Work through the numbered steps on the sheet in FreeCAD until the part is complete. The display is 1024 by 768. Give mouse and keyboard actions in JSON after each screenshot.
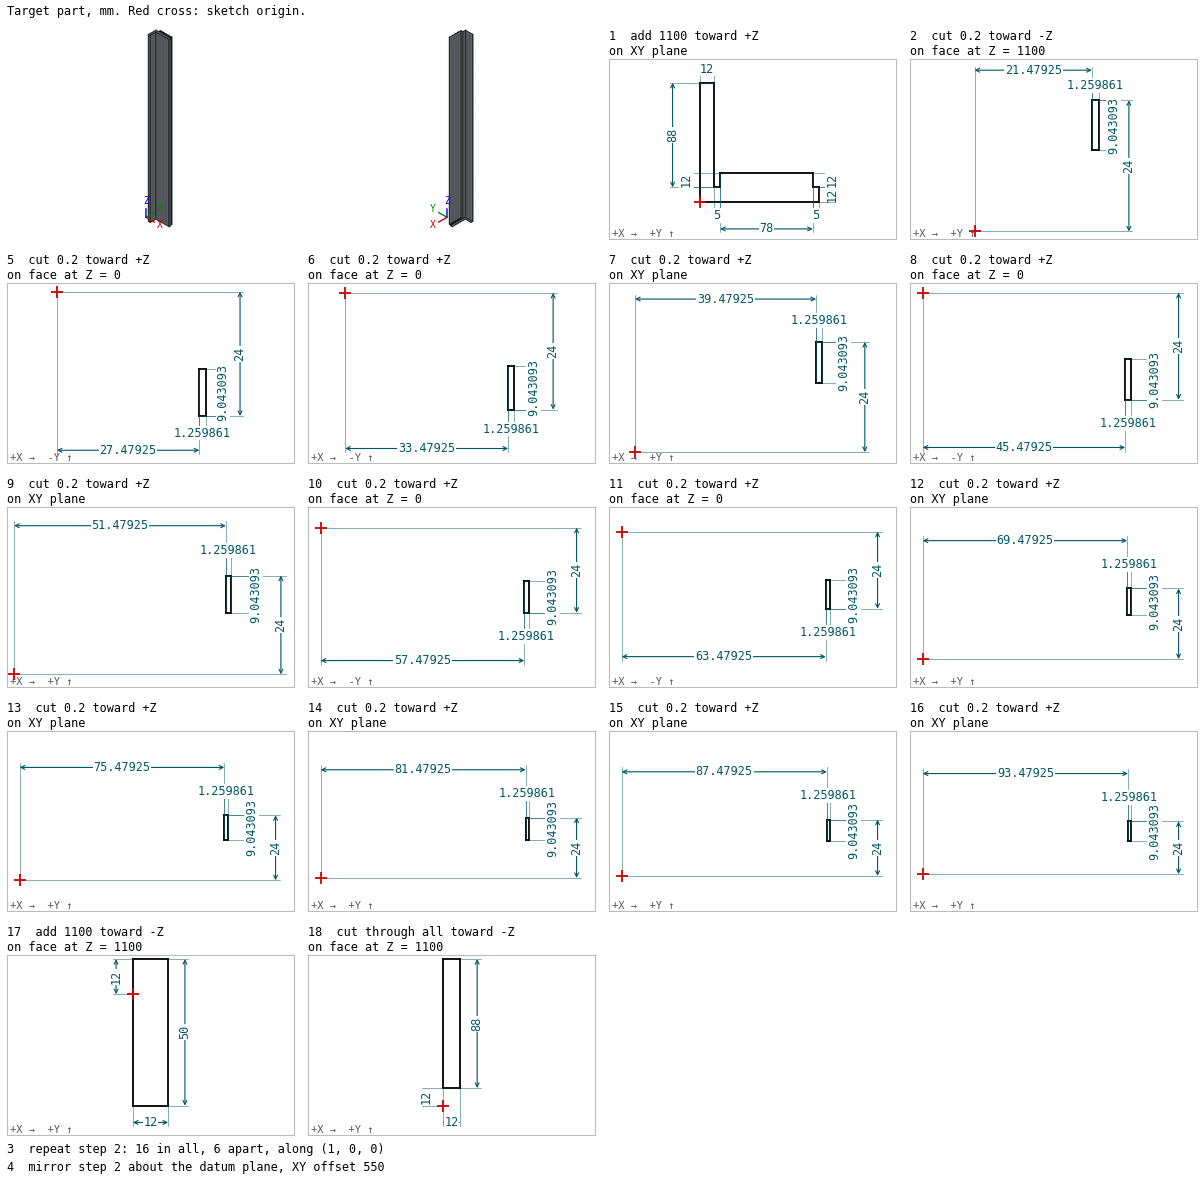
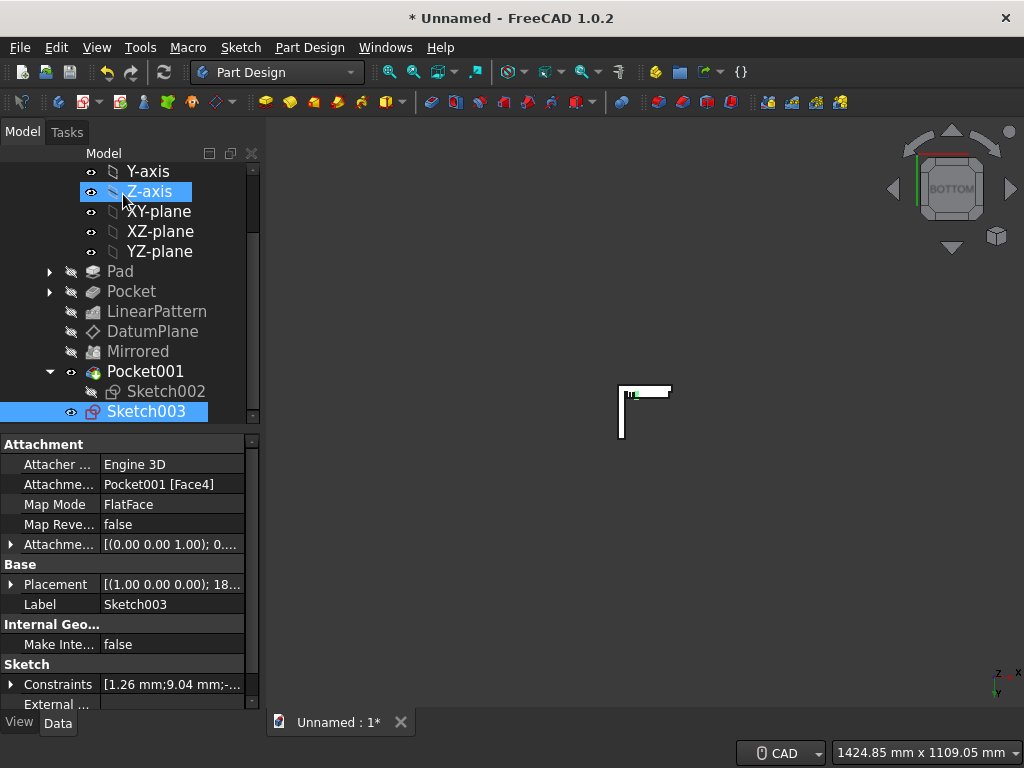
{"action": "left_click", "coordinate": [432, 102]}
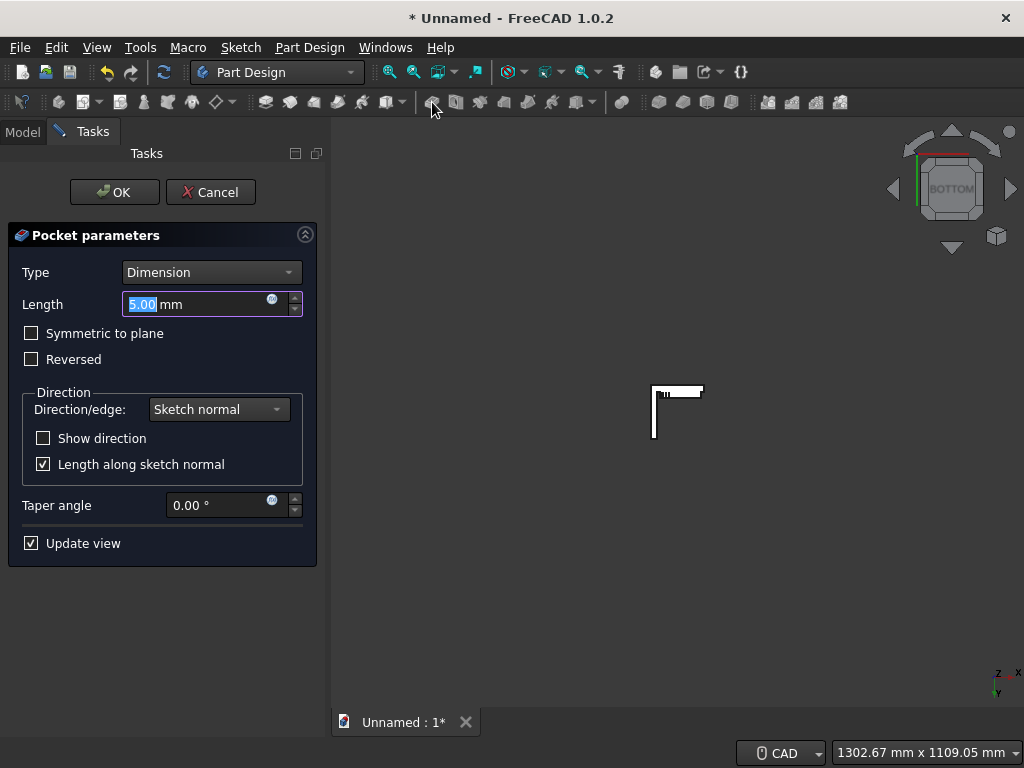
{"action": "type", "text": "0.2"}
{"action": "key", "text": "Tab"}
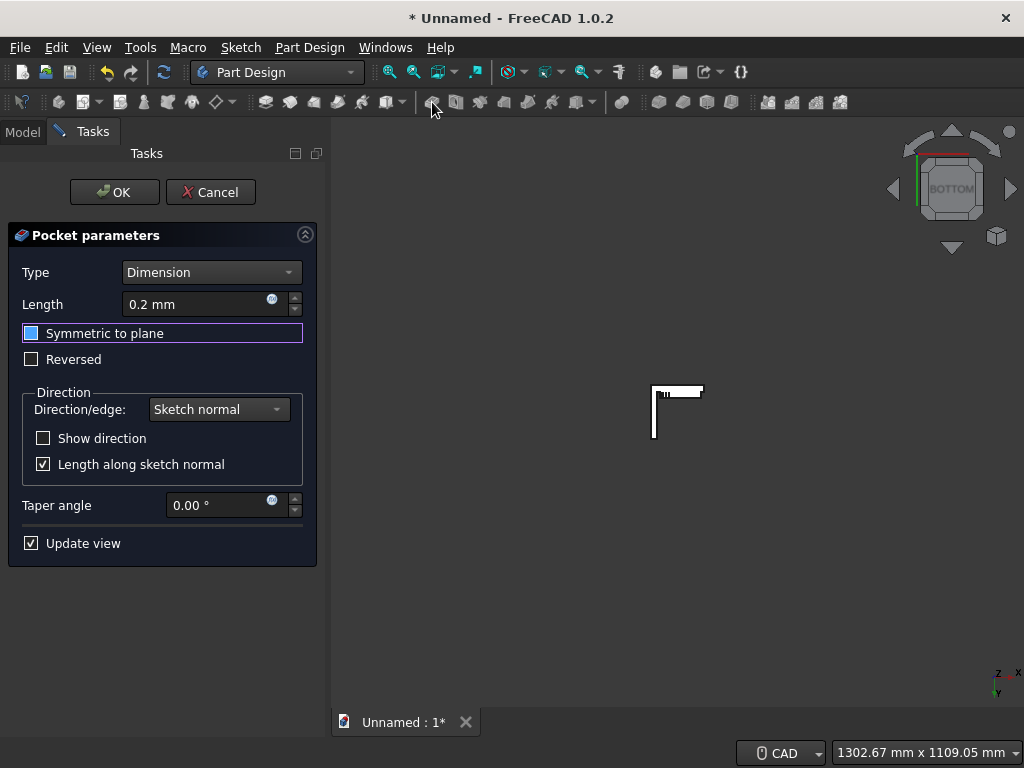
{"action": "left_click", "coordinate": [115, 192]}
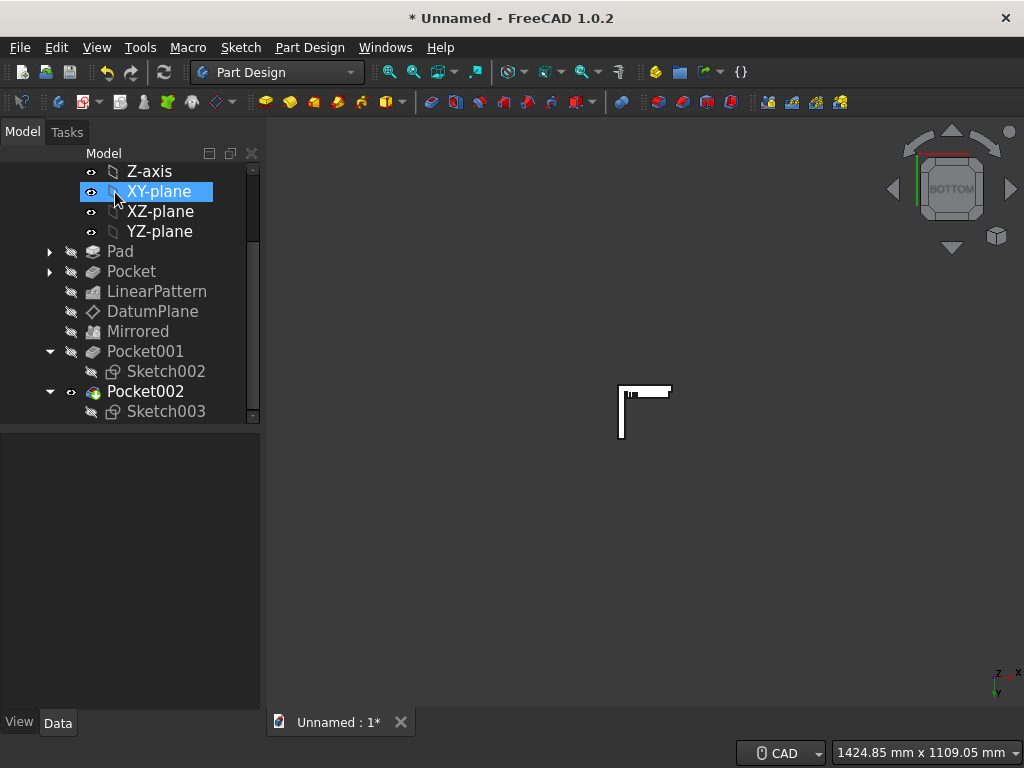
{"action": "left_click", "coordinate": [390, 72]}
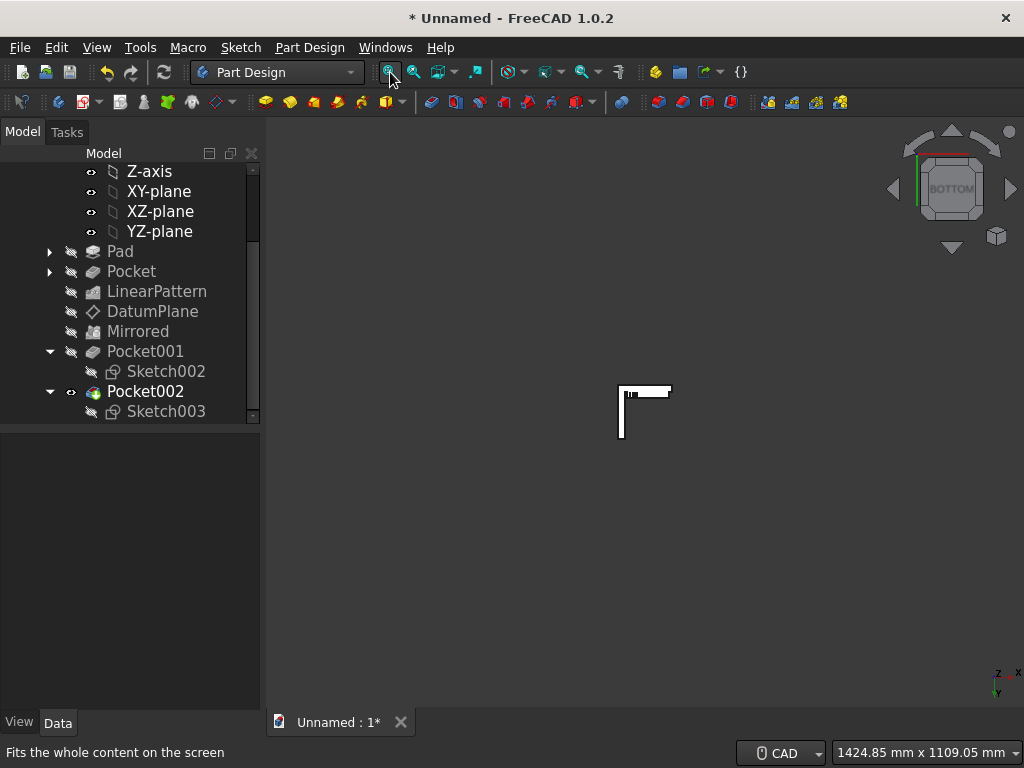
{"action": "left_click", "coordinate": [84, 102]}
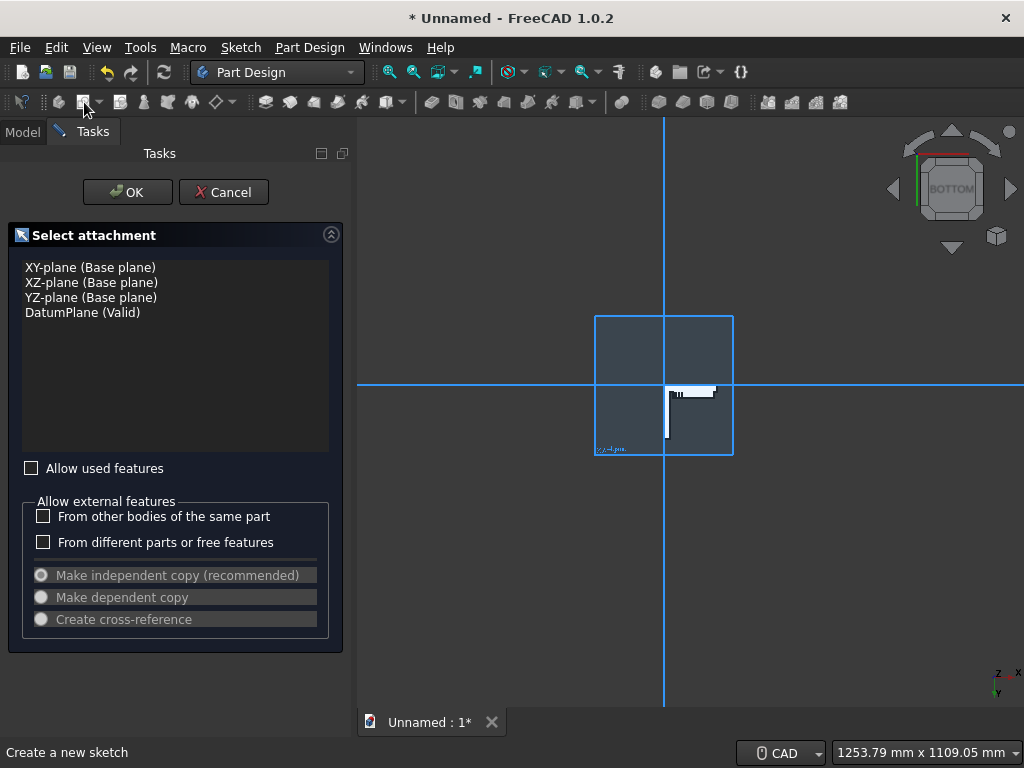
{"action": "left_click", "coordinate": [82, 268]}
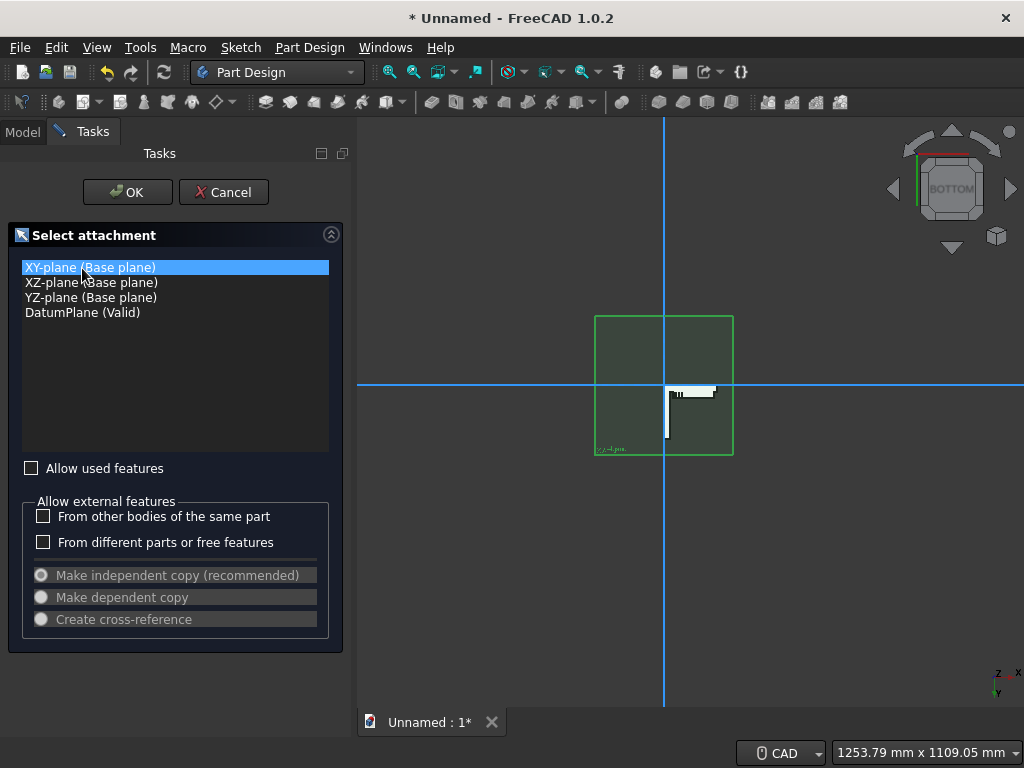
{"action": "left_click", "coordinate": [128, 192]}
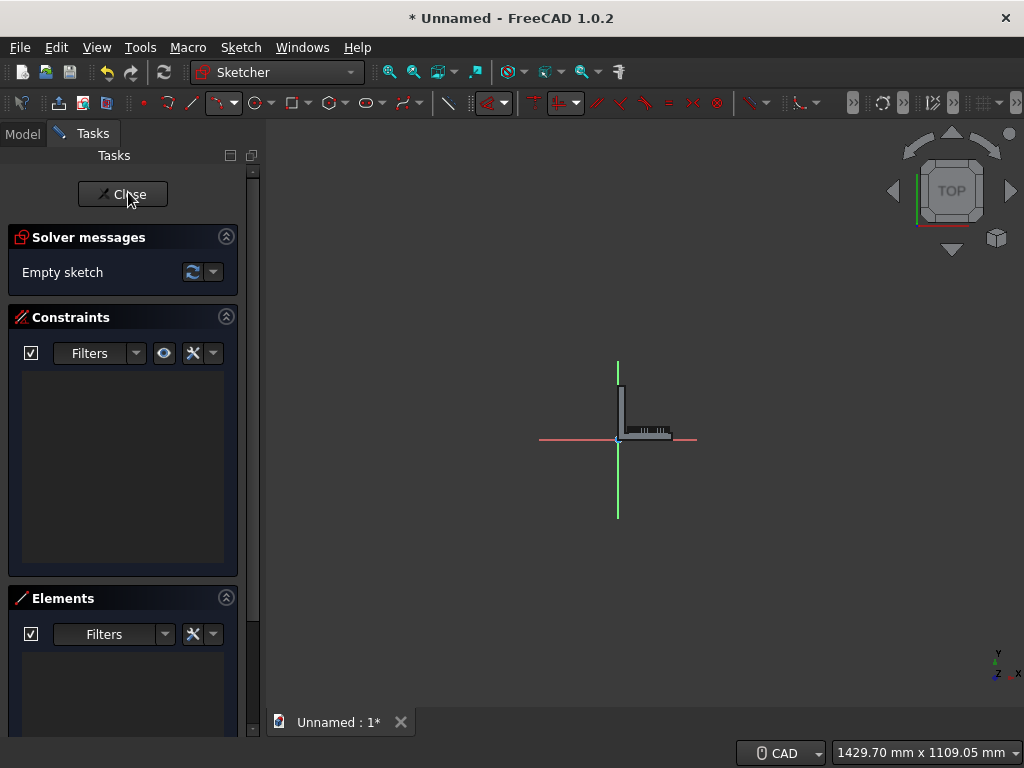
{"action": "left_click", "coordinate": [108, 104]}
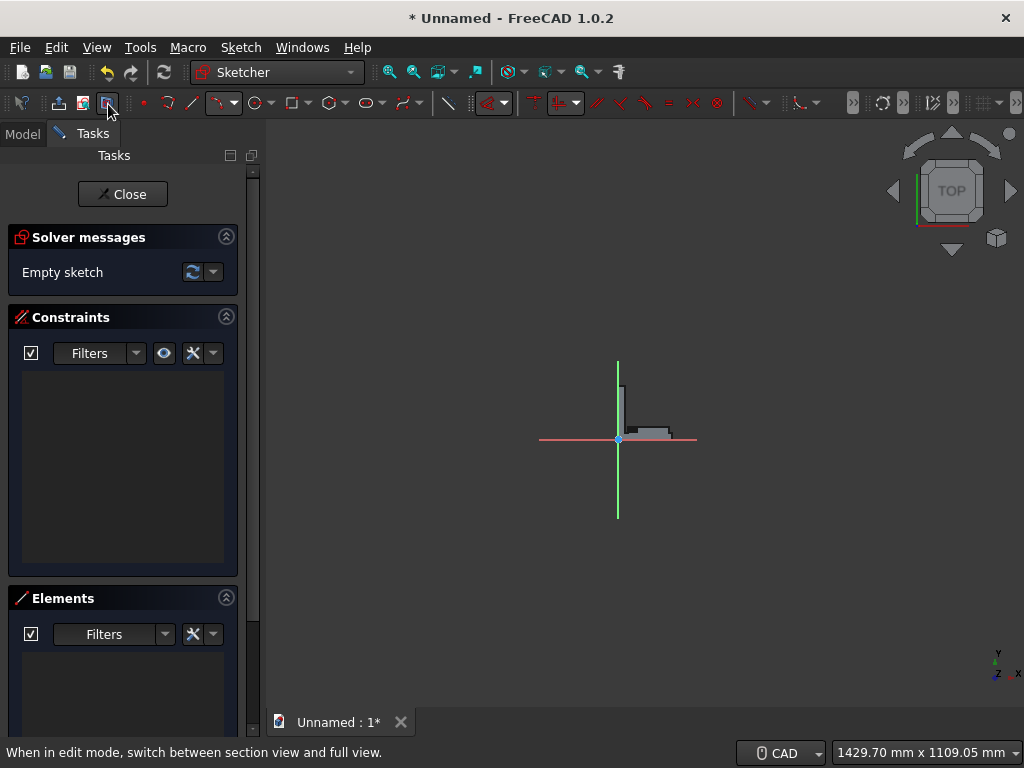
{"action": "scroll", "coordinate": [643, 430], "scroll_direction": "up", "scroll_amount": 15}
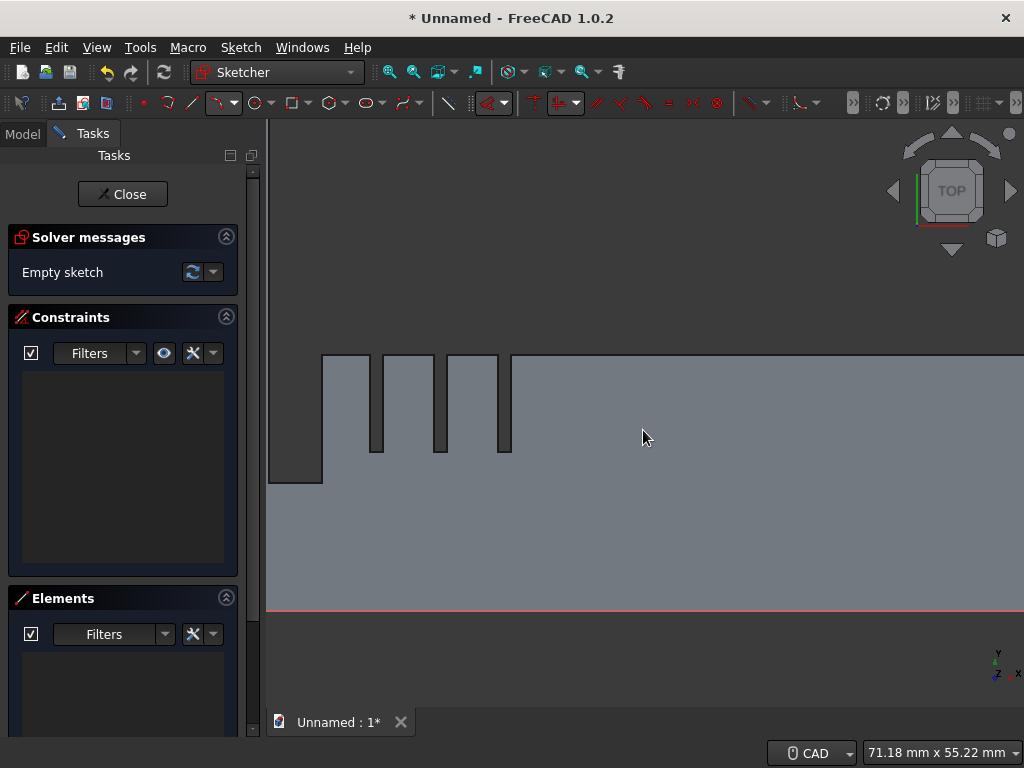
{"action": "scroll", "coordinate": [566, 400], "scroll_direction": "up", "scroll_amount": 7}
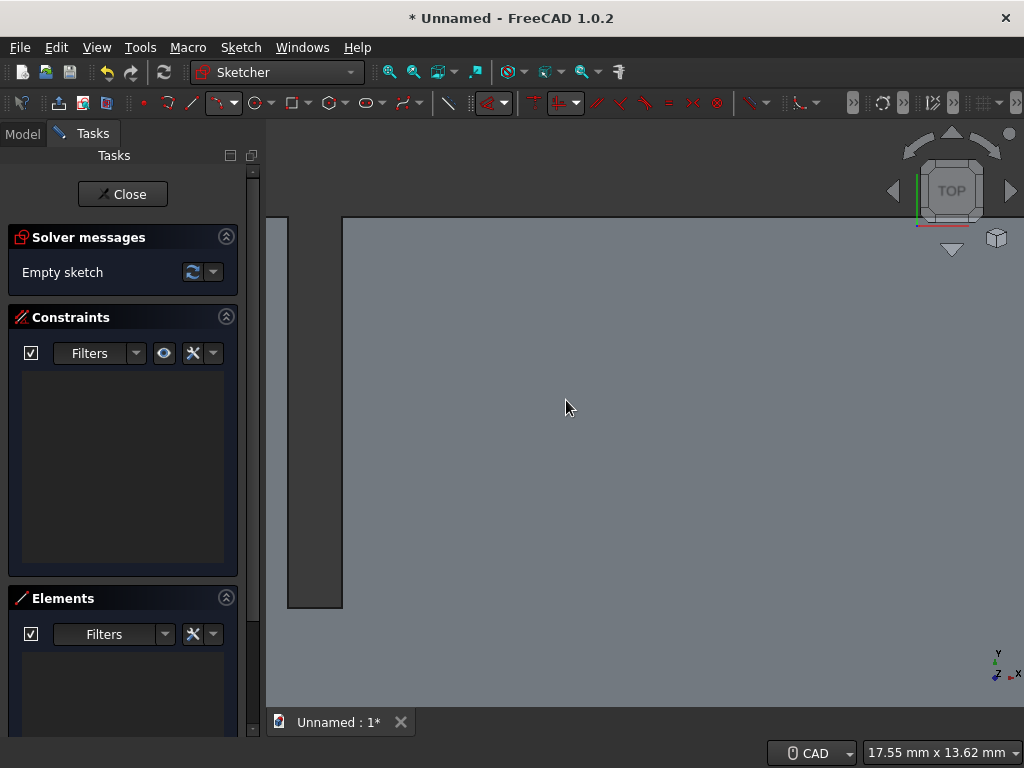
{"action": "left_click", "coordinate": [292, 104]}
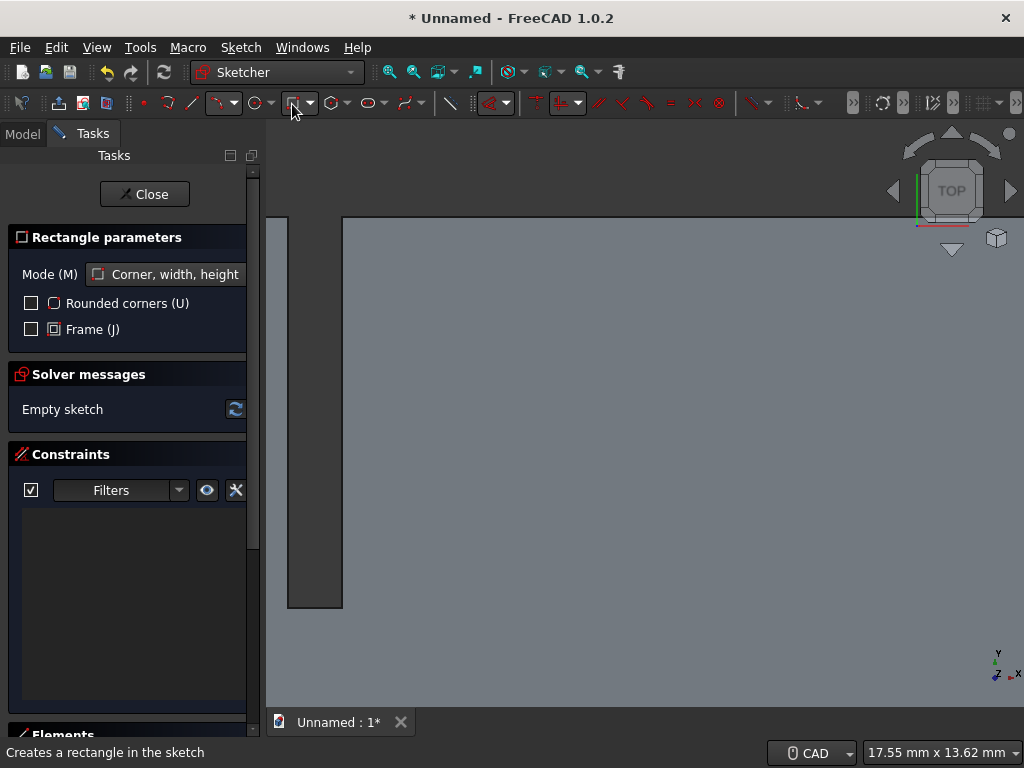
{"action": "left_click", "coordinate": [547, 217]}
{"action": "mouse_move", "coordinate": [601, 608]}